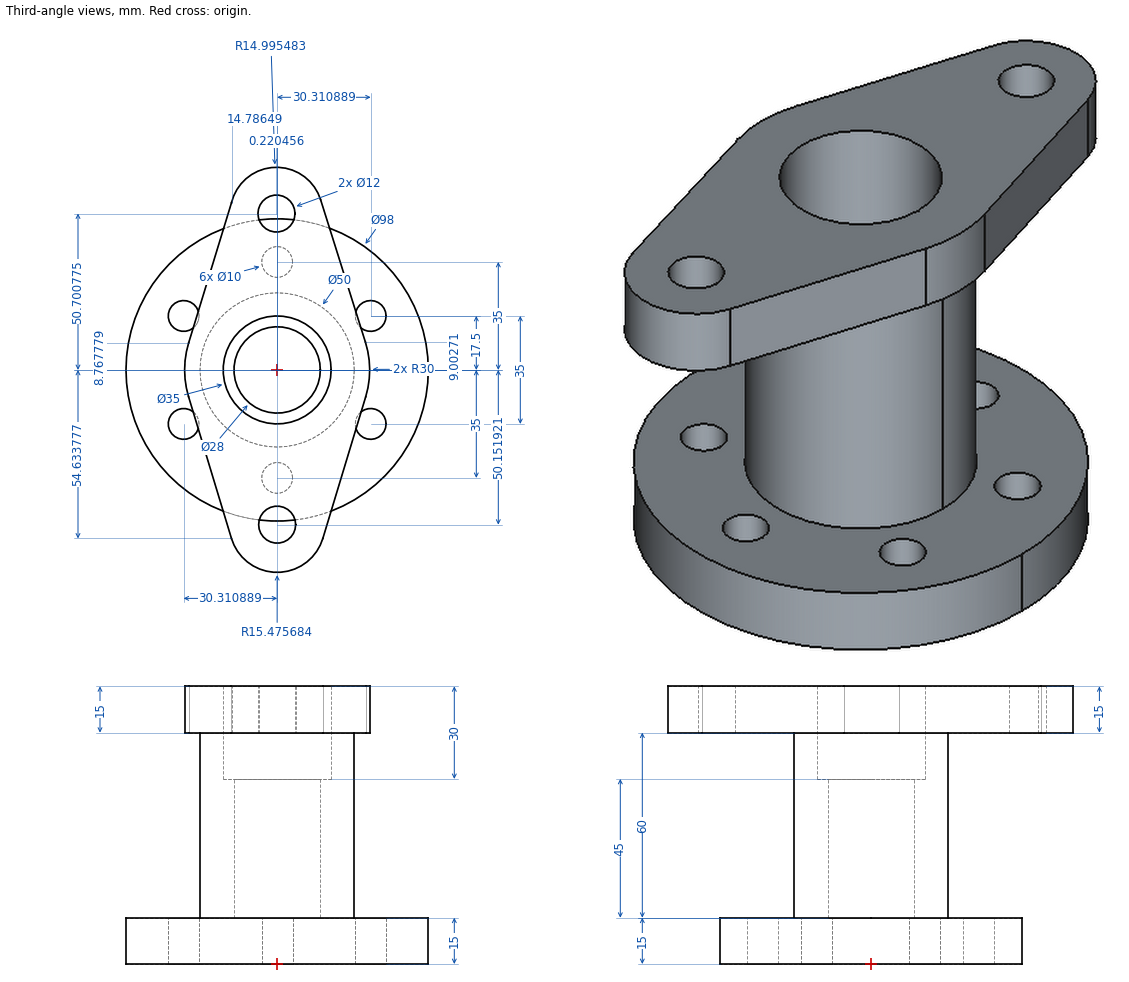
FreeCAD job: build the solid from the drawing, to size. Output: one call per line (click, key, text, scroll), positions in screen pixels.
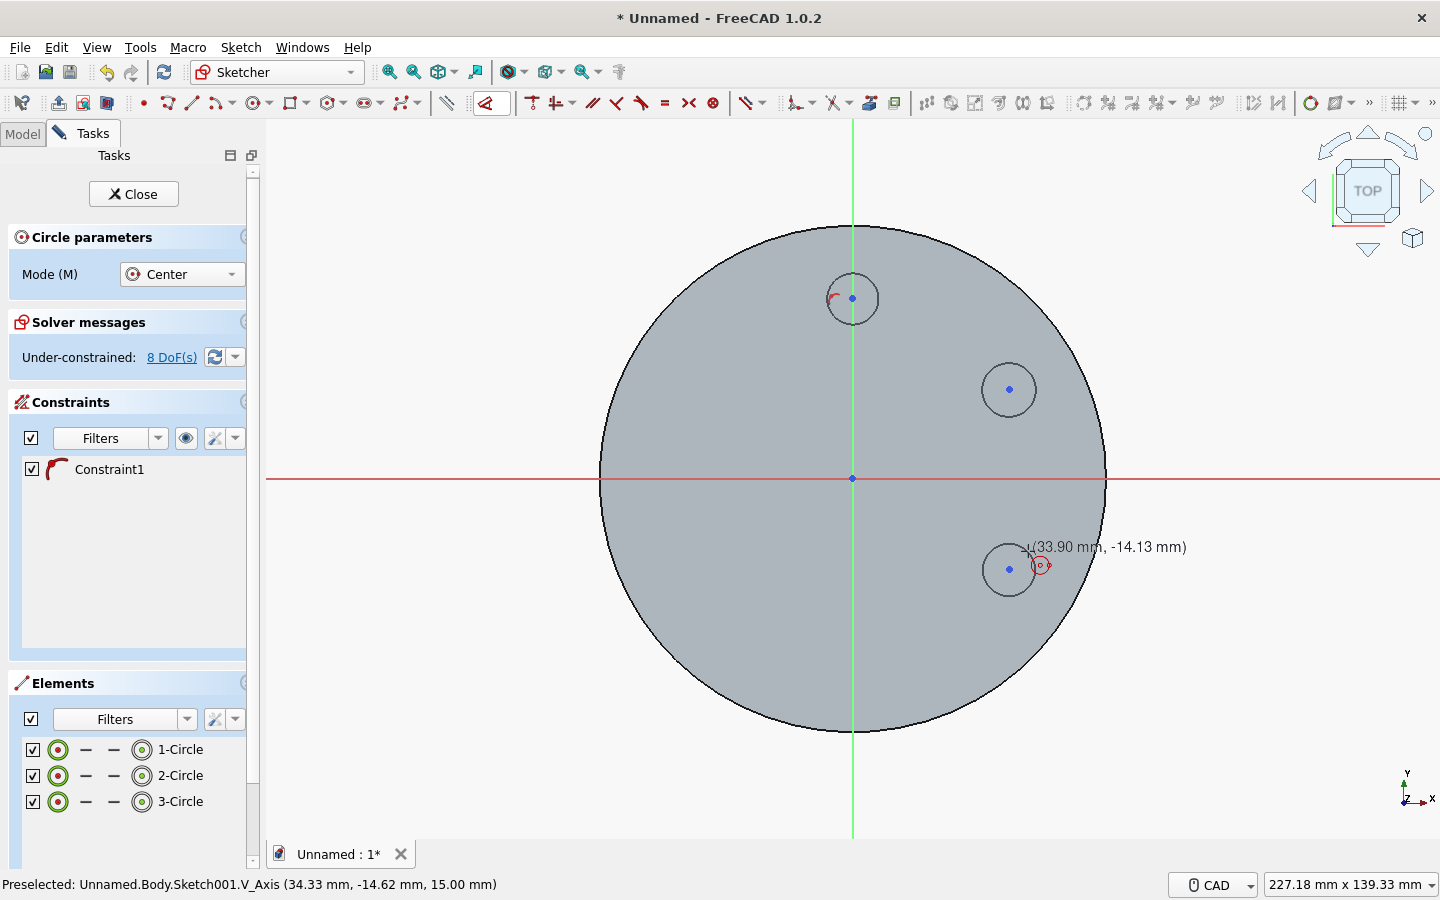
click(853, 660)
click(871, 642)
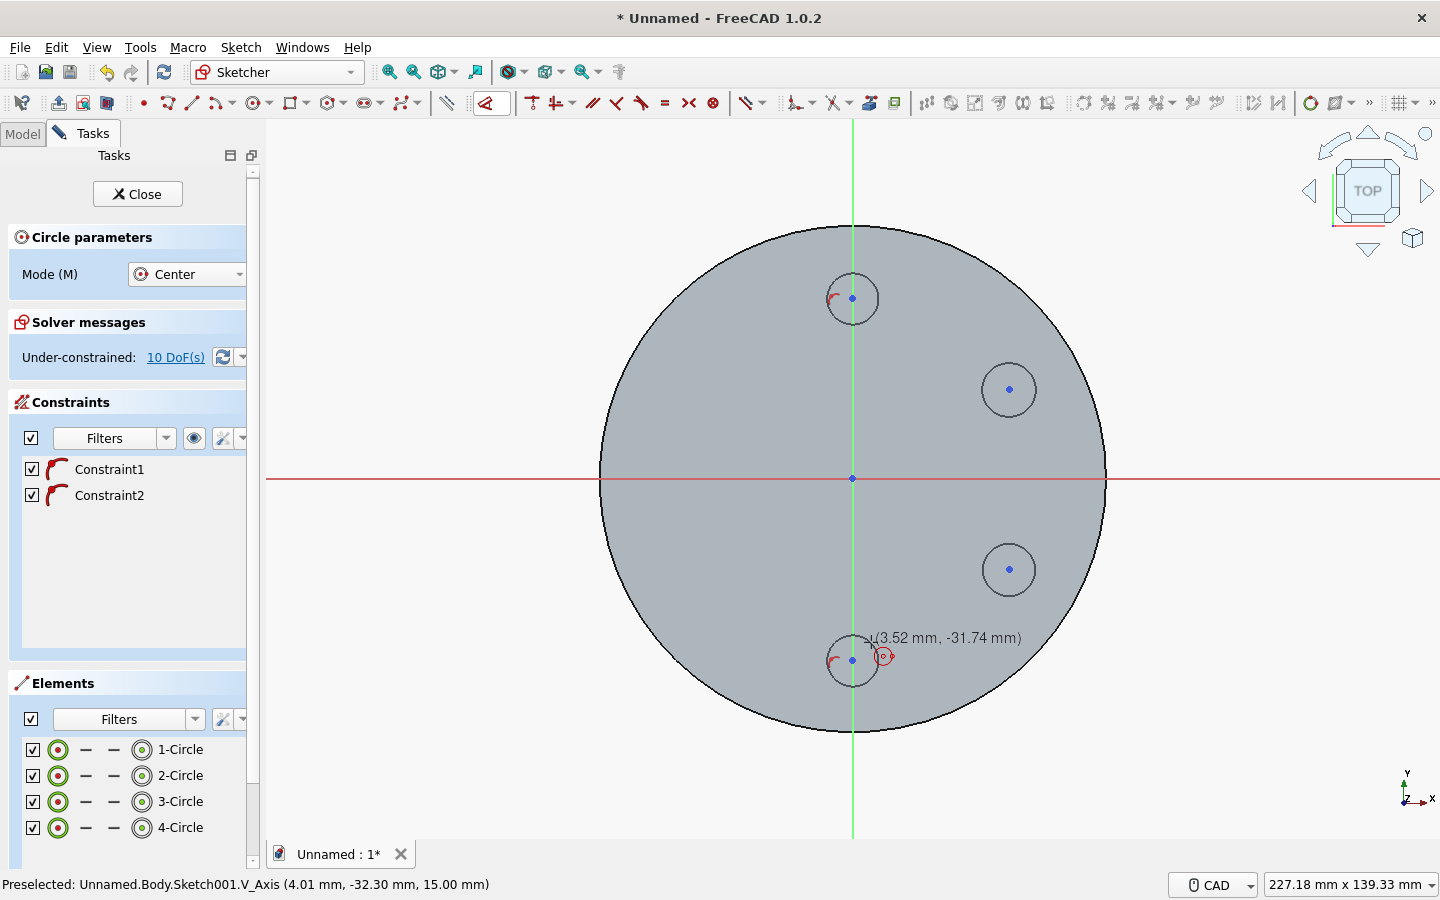
click(696, 569)
click(714, 551)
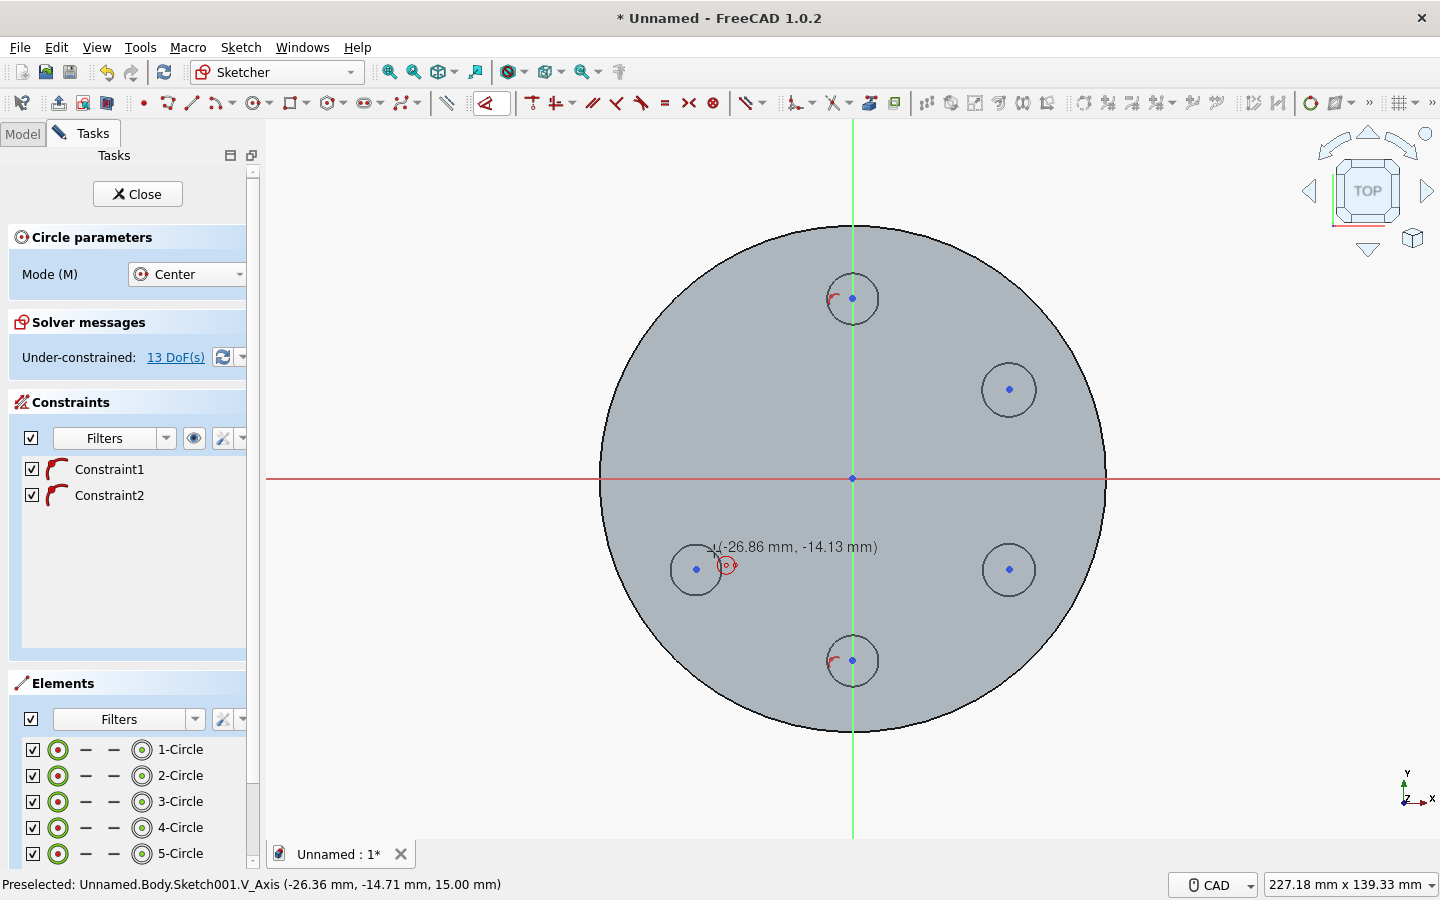
click(696, 389)
click(714, 370)
key(Escape)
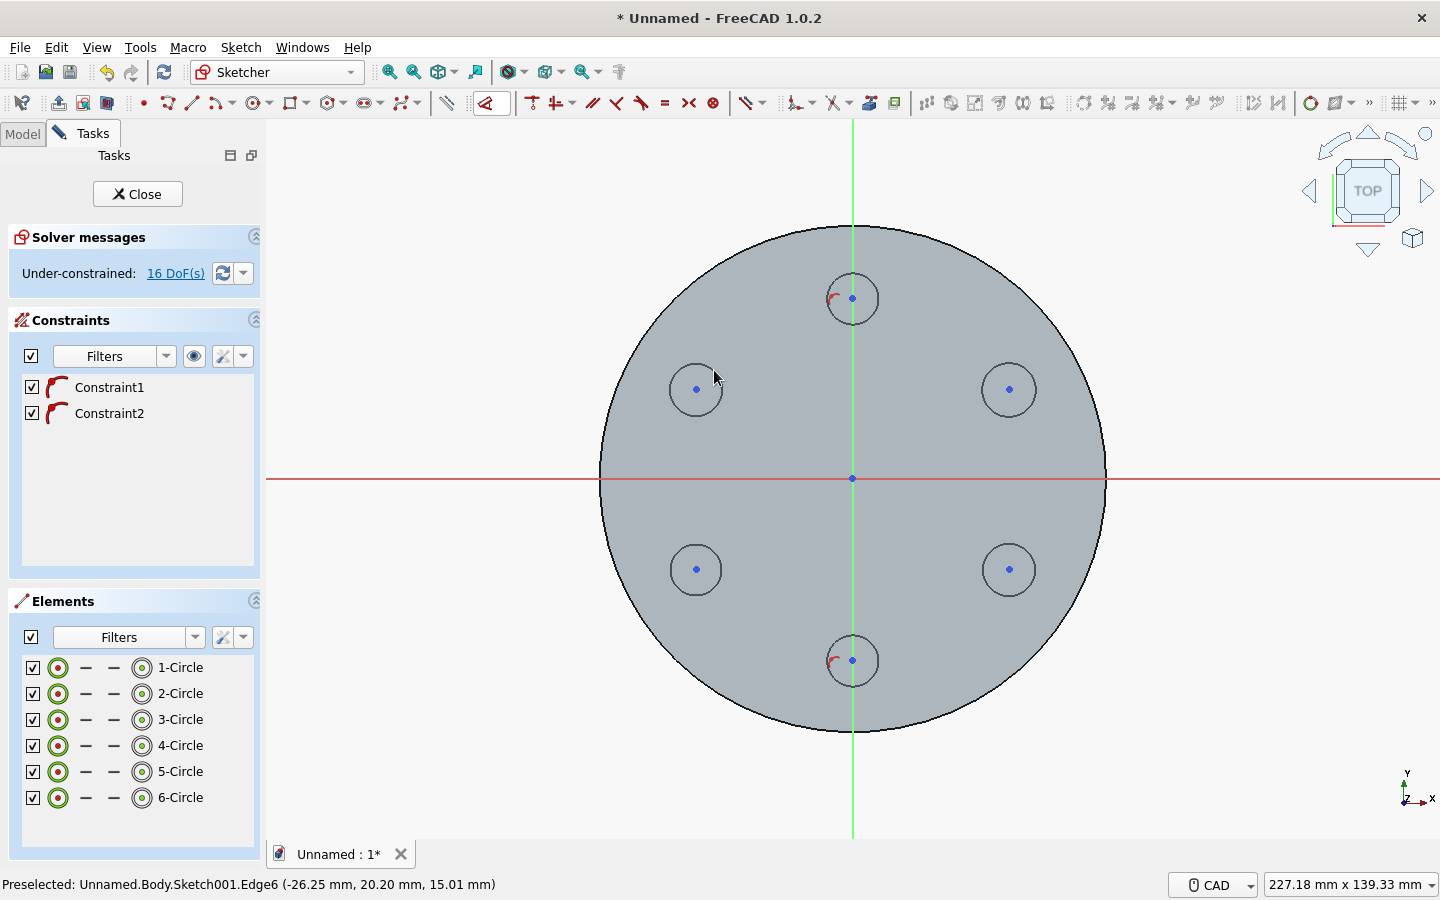
click(871, 281)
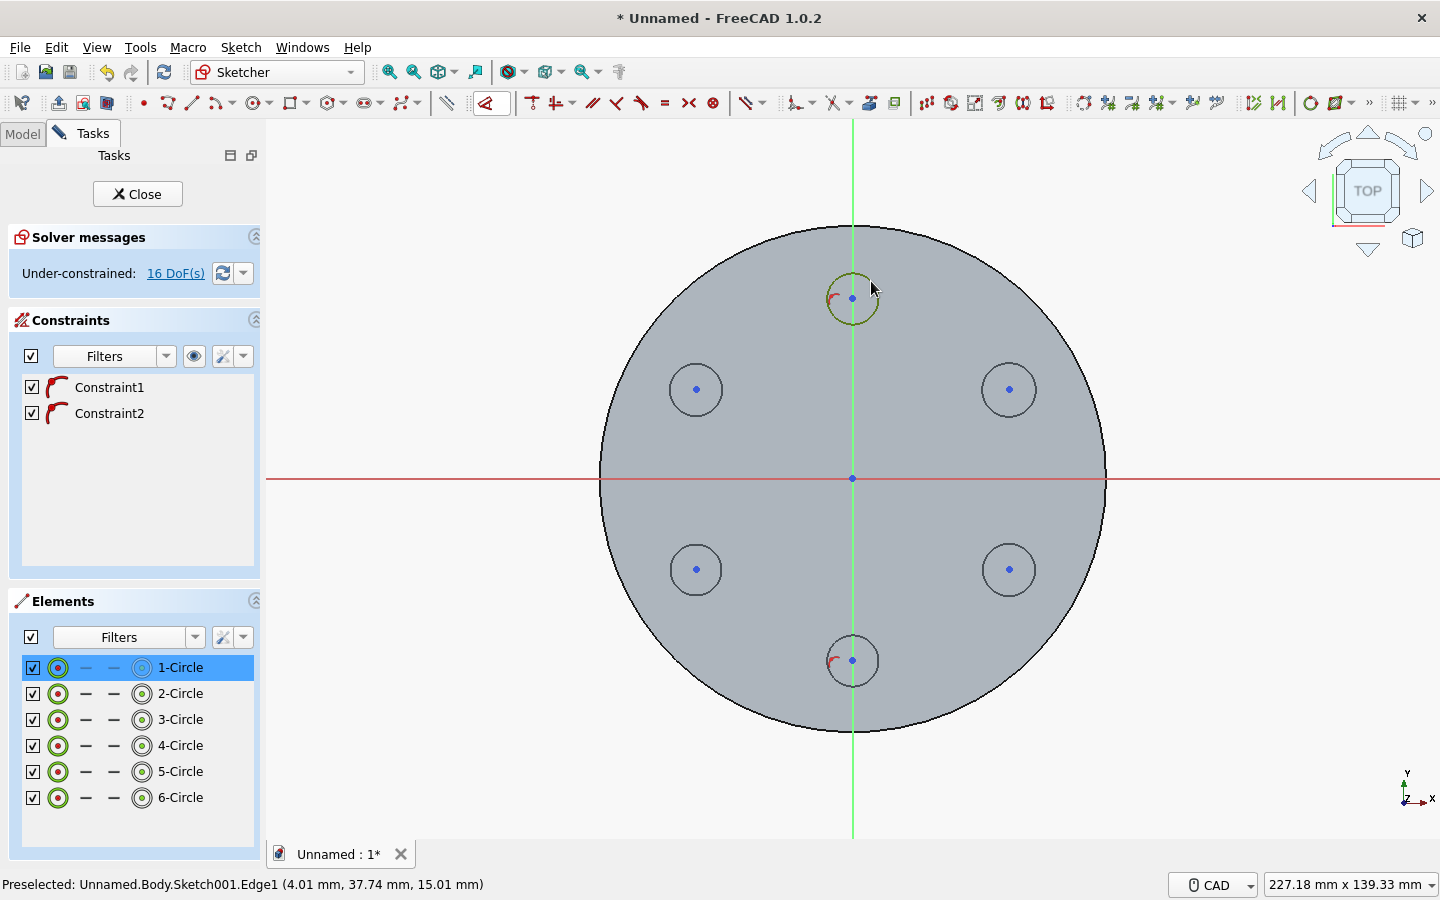
click(1028, 371)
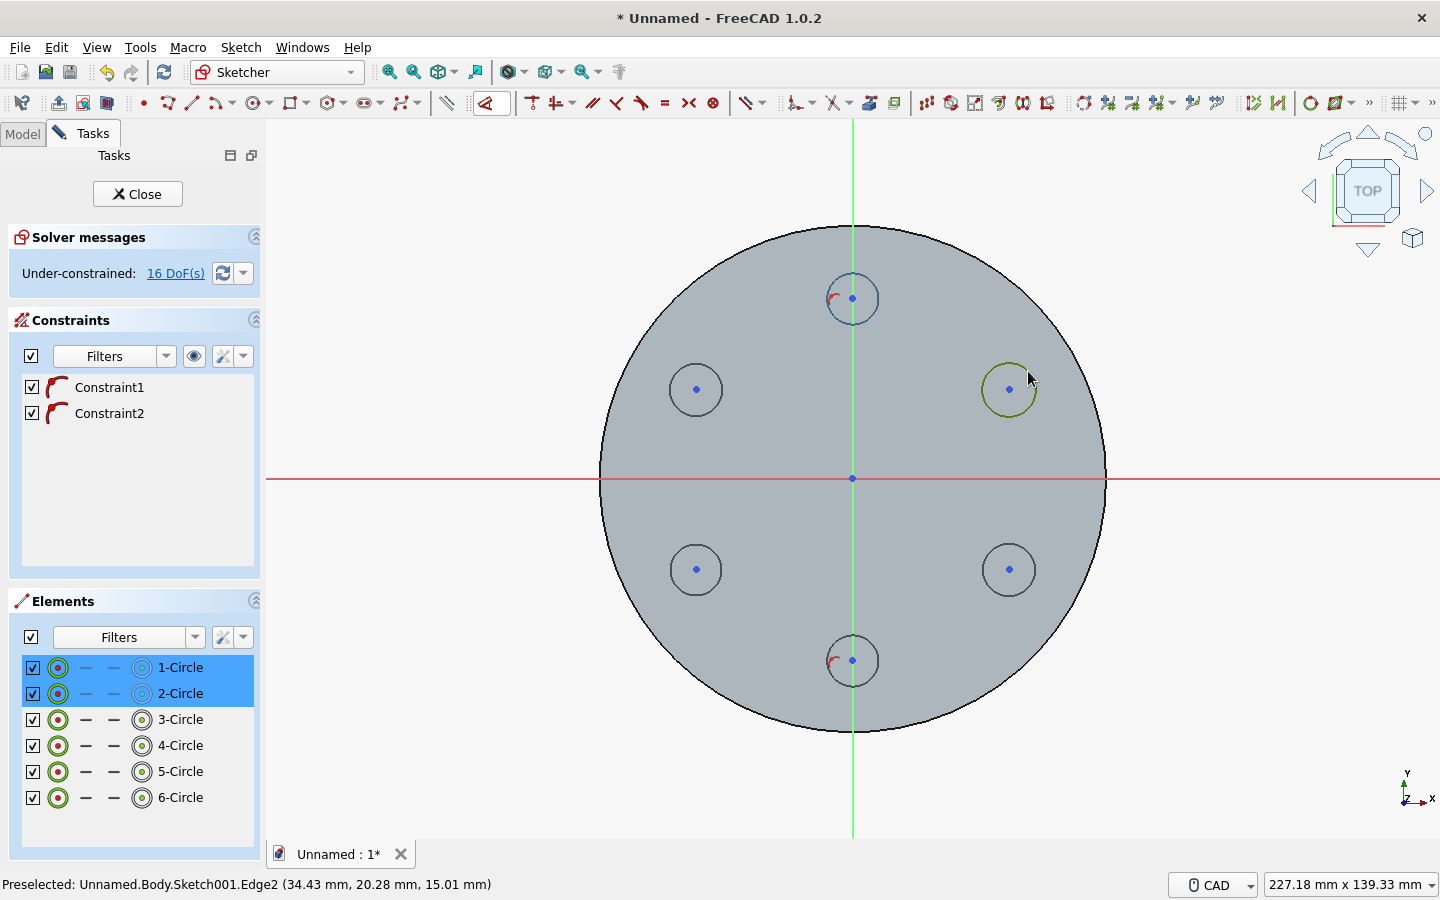
click(1027, 551)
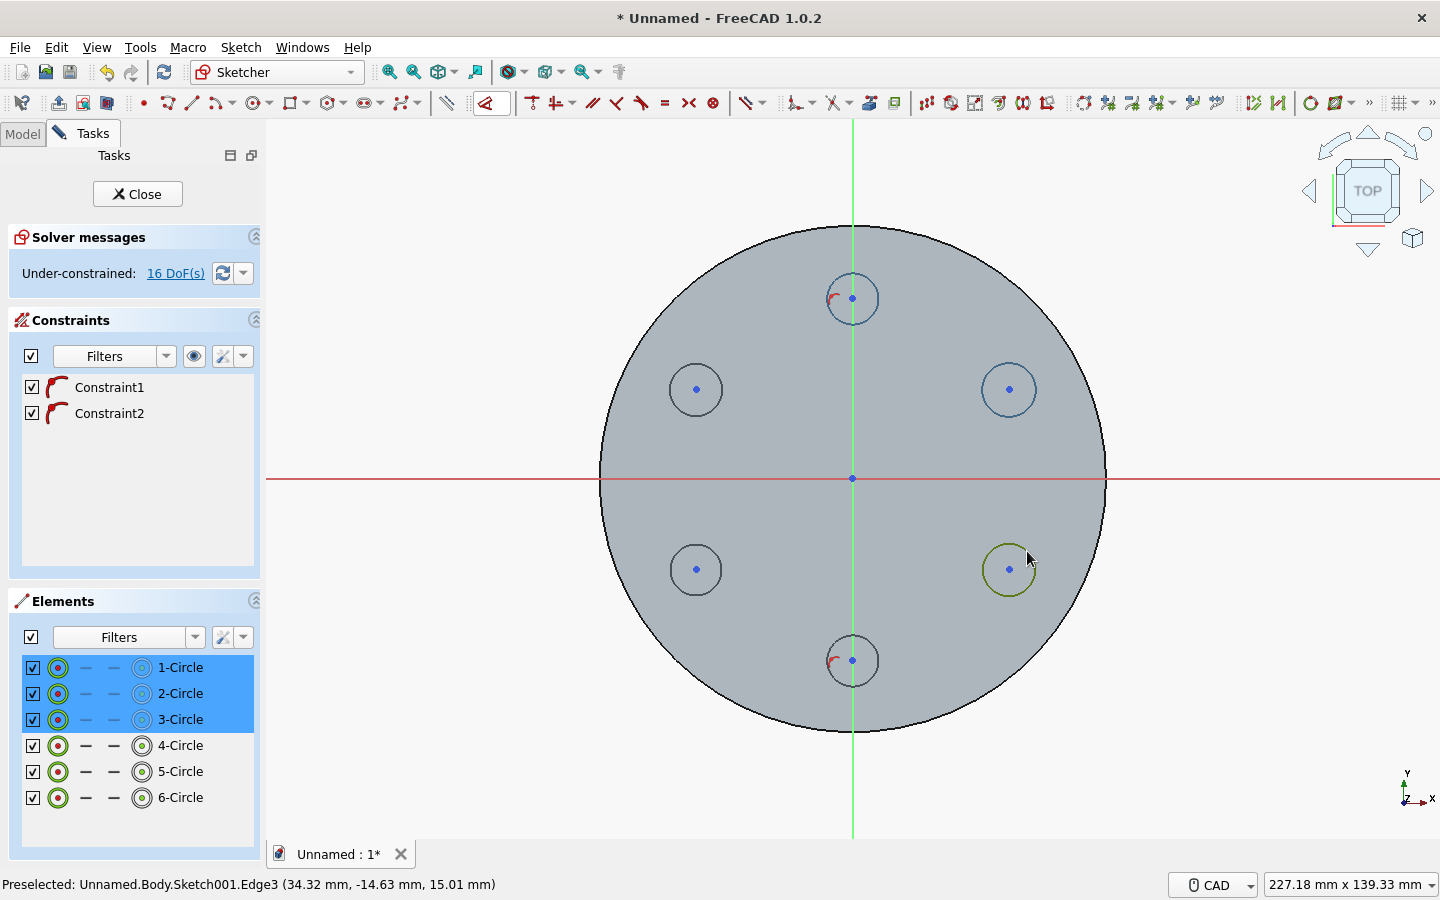
click(871, 643)